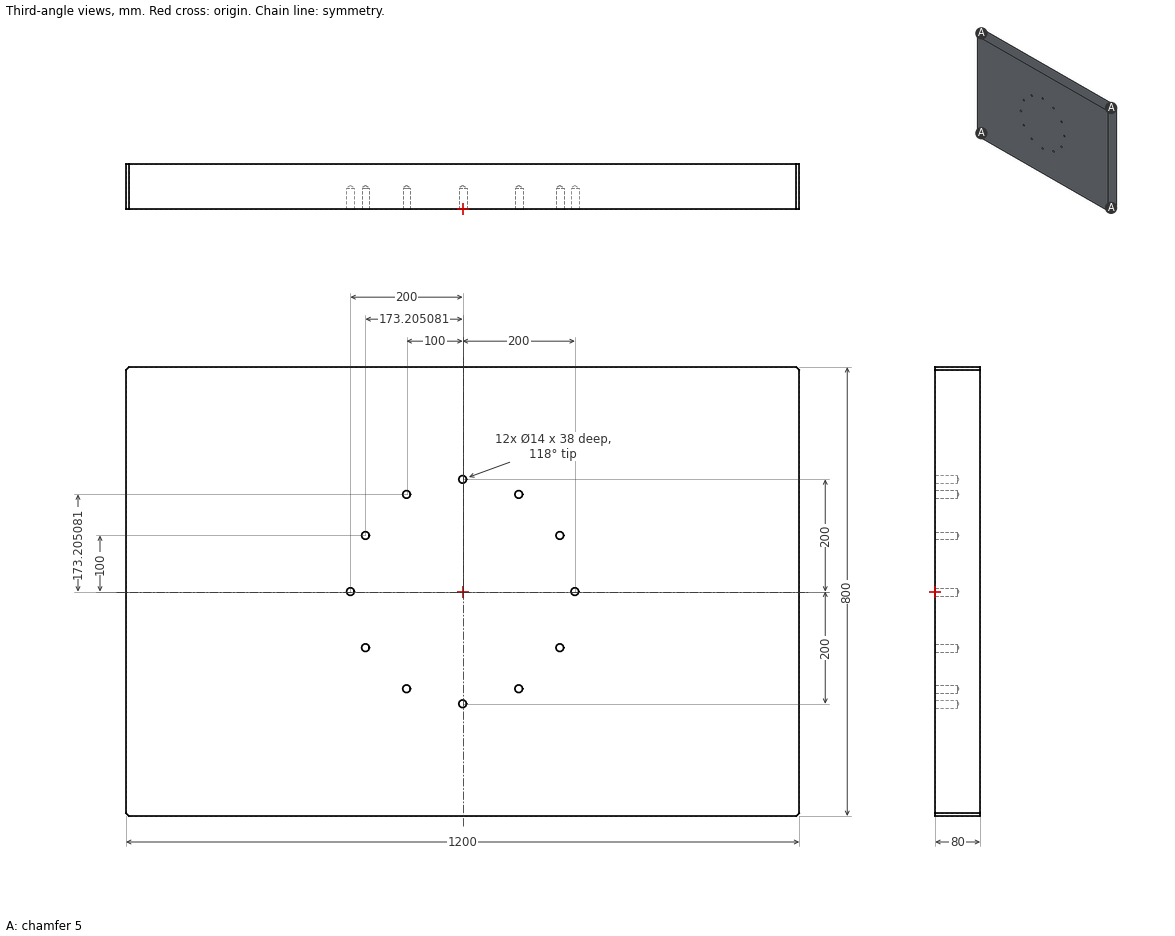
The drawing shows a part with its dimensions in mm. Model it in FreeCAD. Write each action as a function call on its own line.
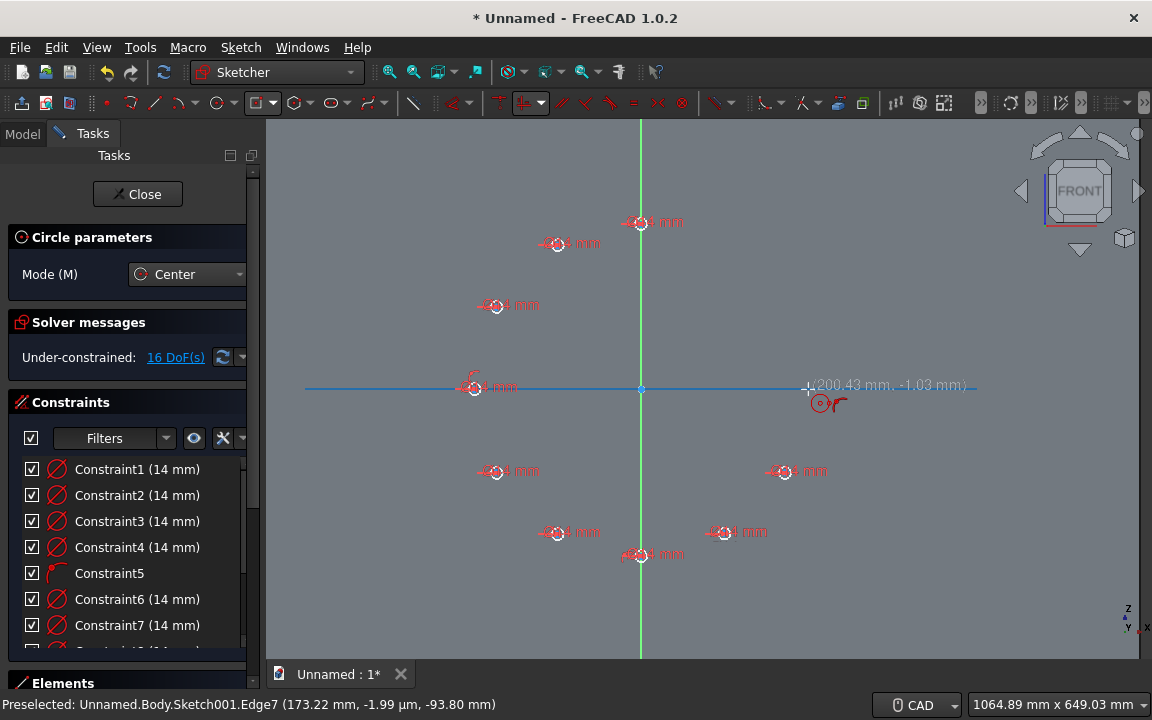
click(808, 389)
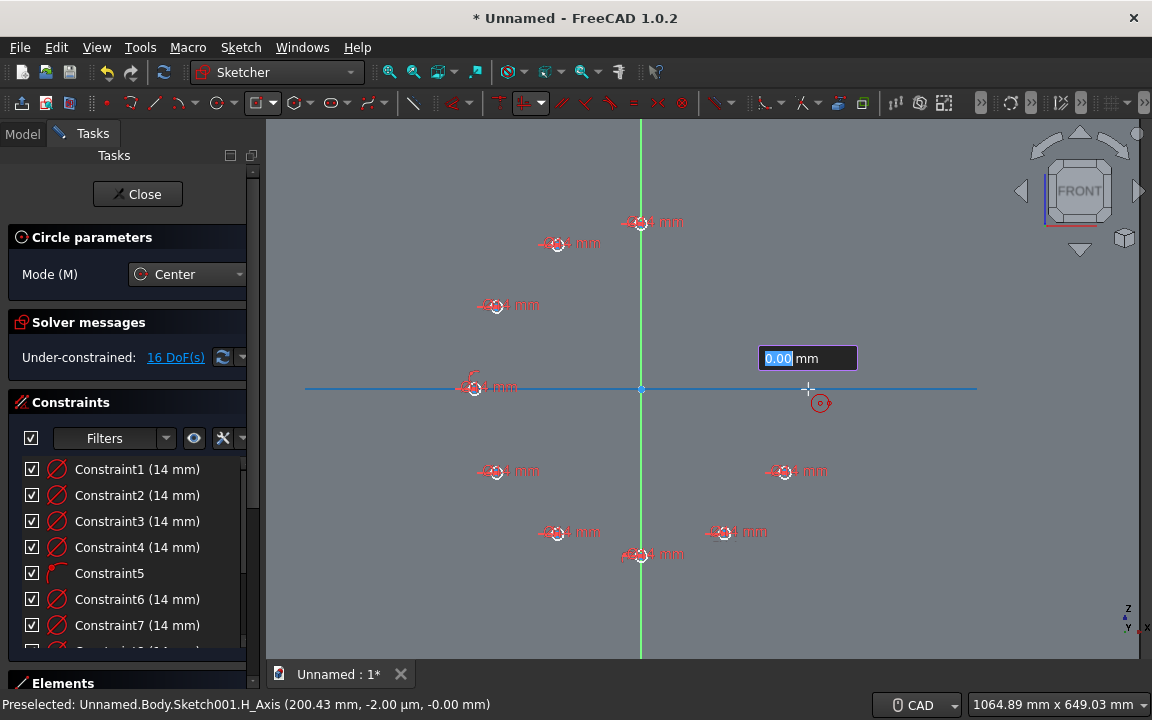
scroll(810, 384, up, 6)
move(807, 382)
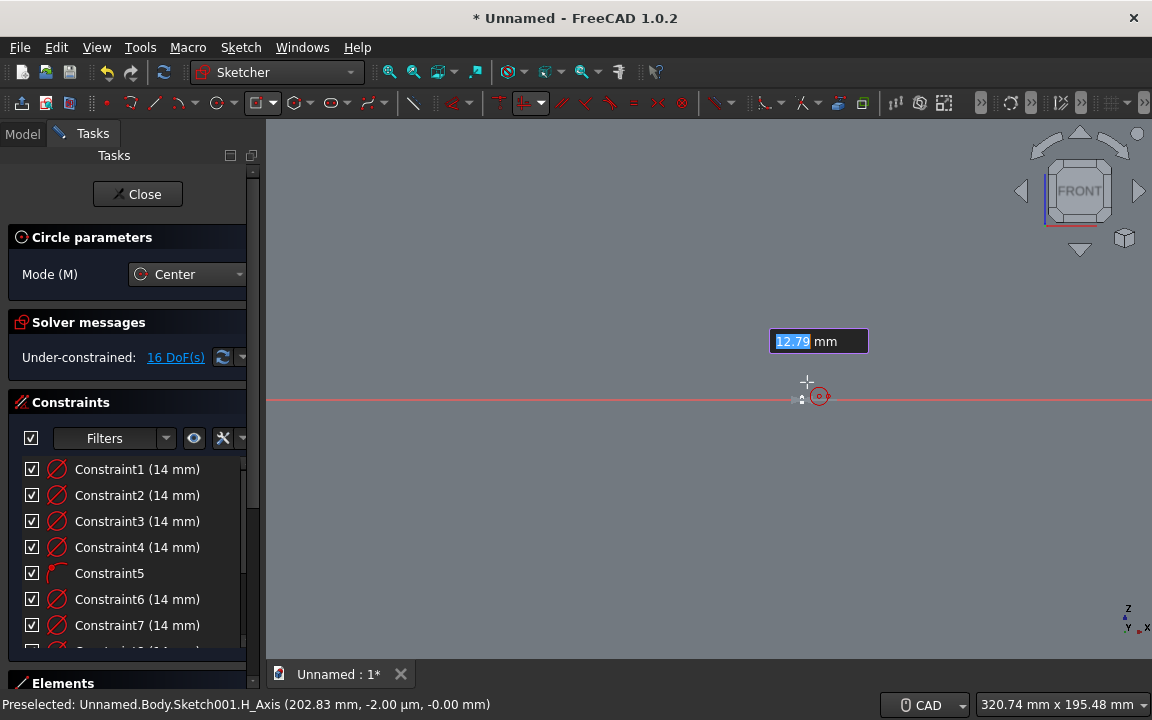
text(14)
key(Return)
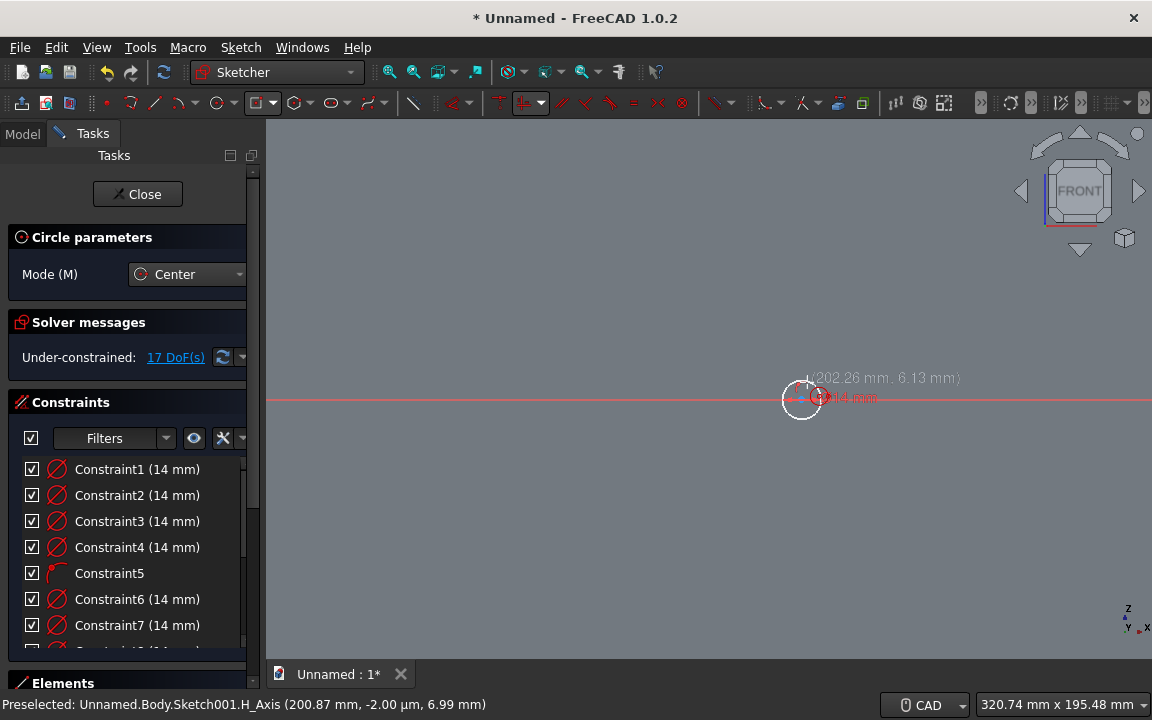
scroll(810, 384, down, 6)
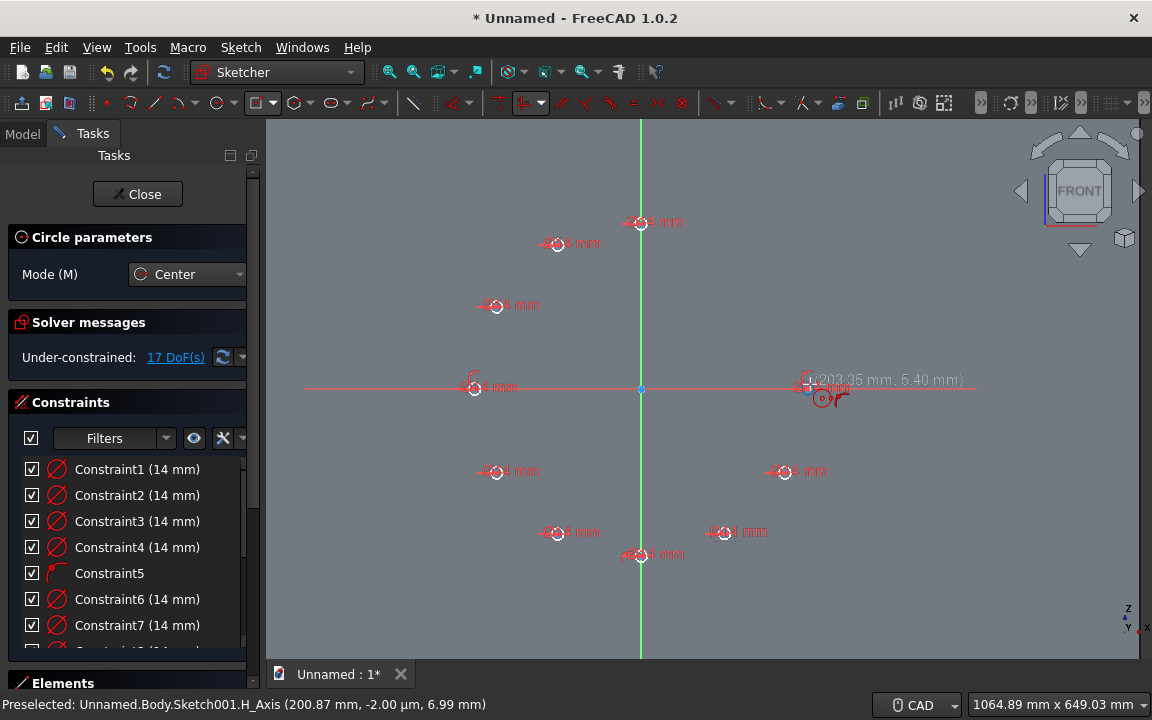
scroll(785, 306, up, 7)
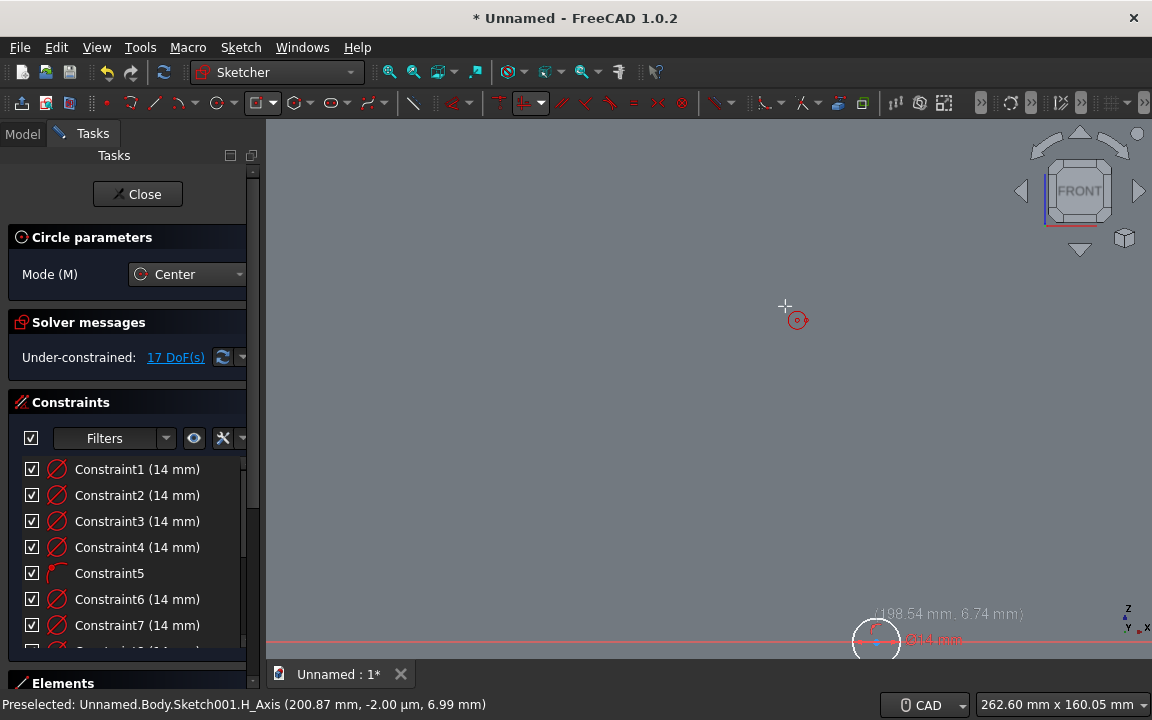
scroll(785, 306, down, 7)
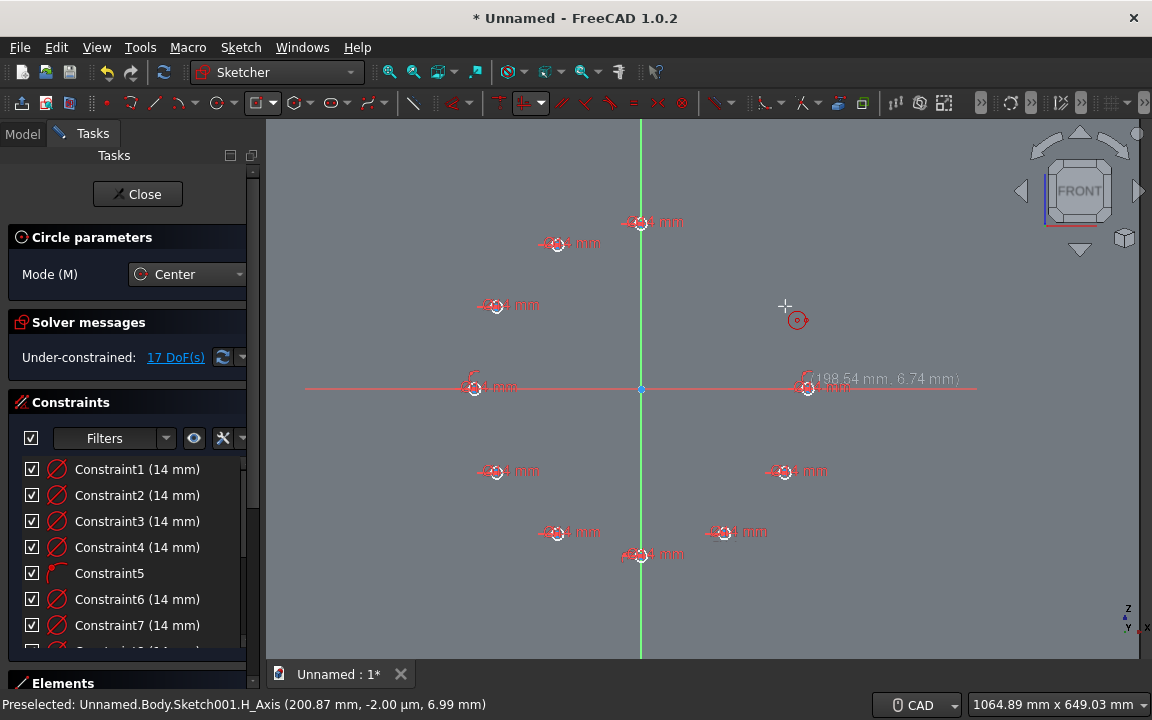
click(785, 306)
move(789, 302)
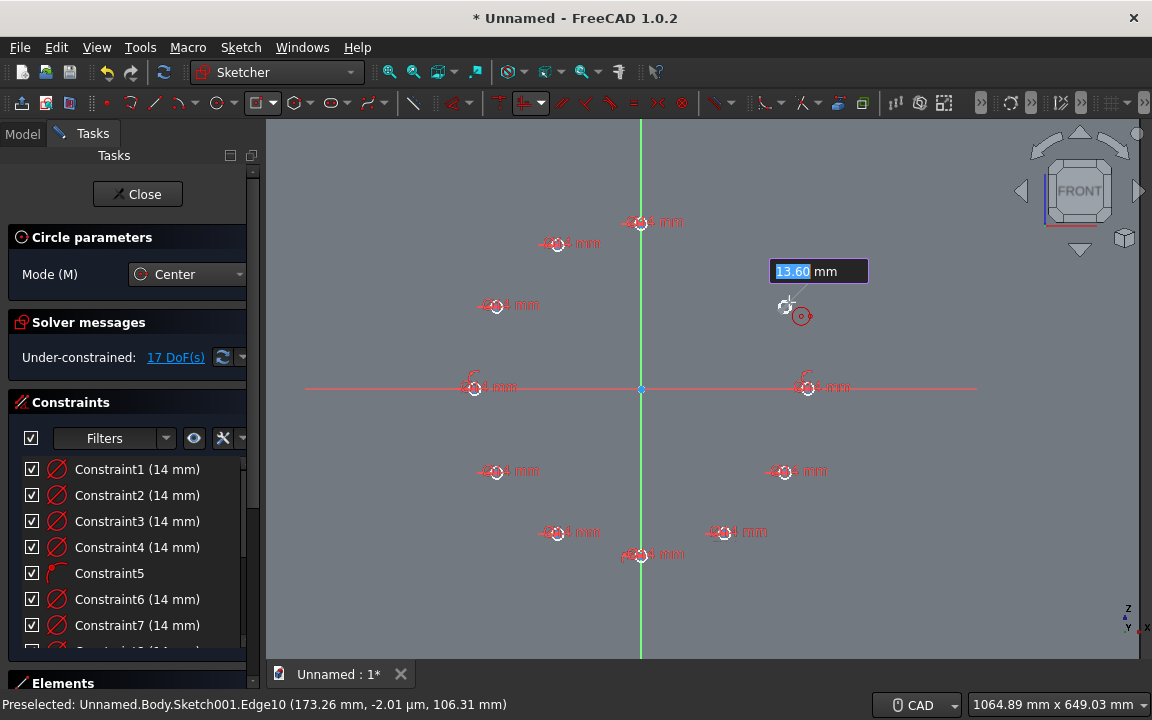
text(14)
key(Return)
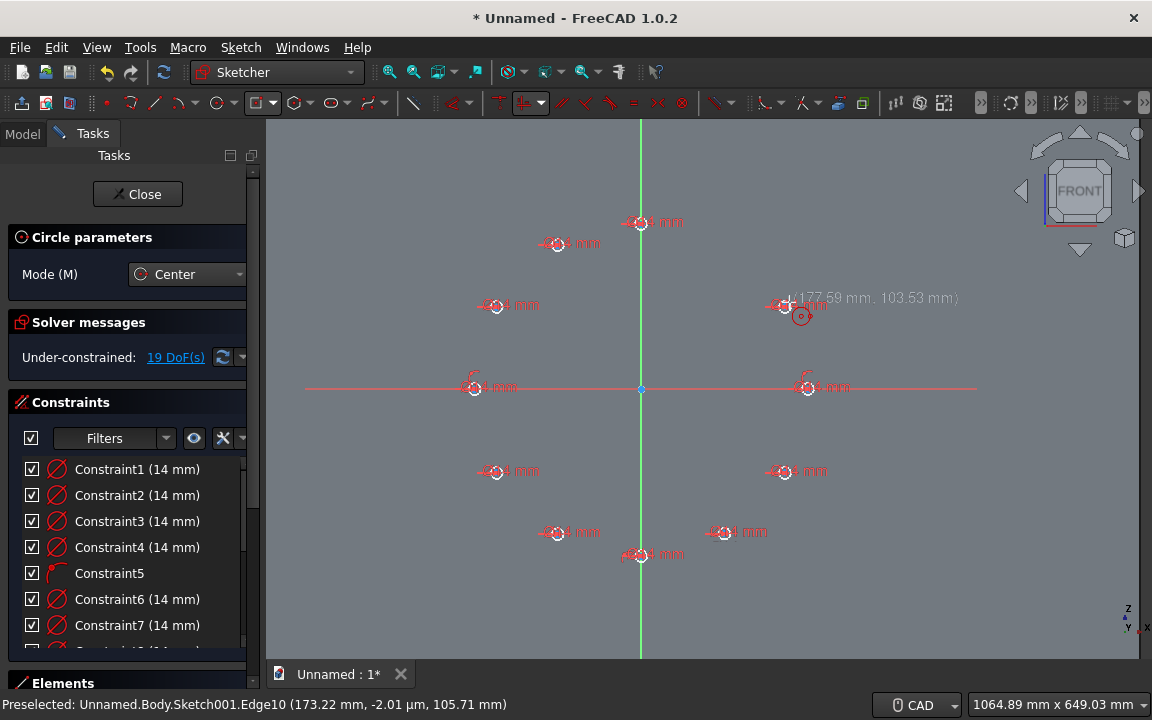
scroll(724, 245, up, 7)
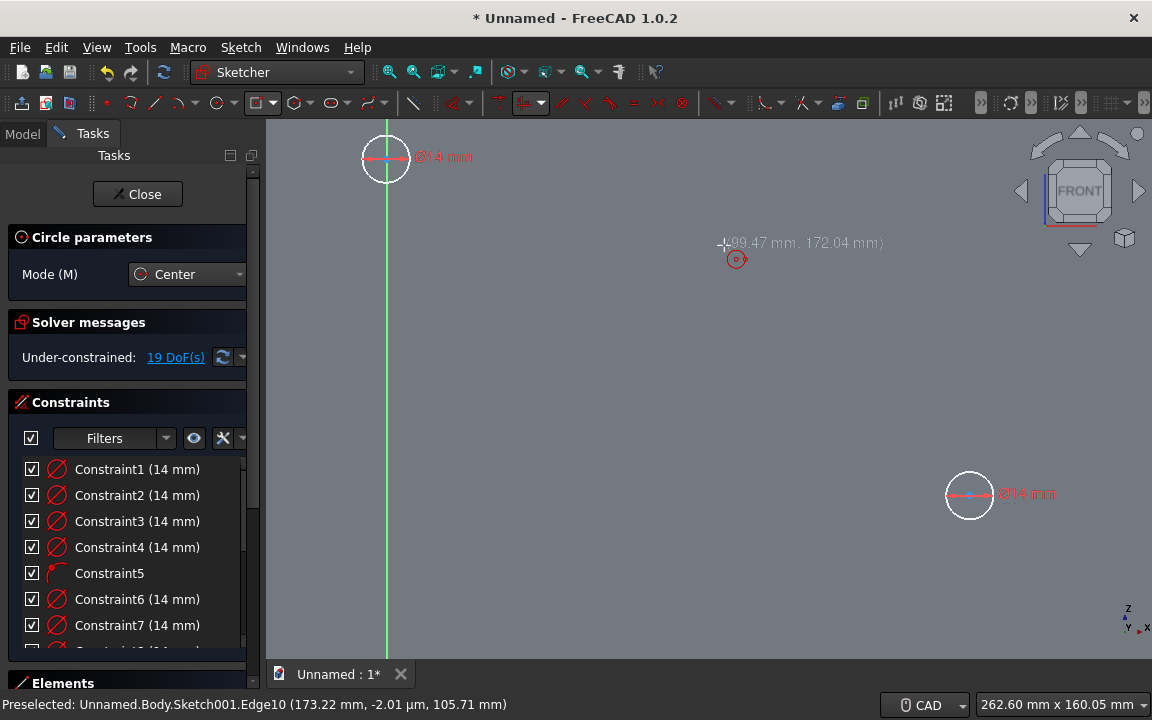
scroll(724, 245, down, 7)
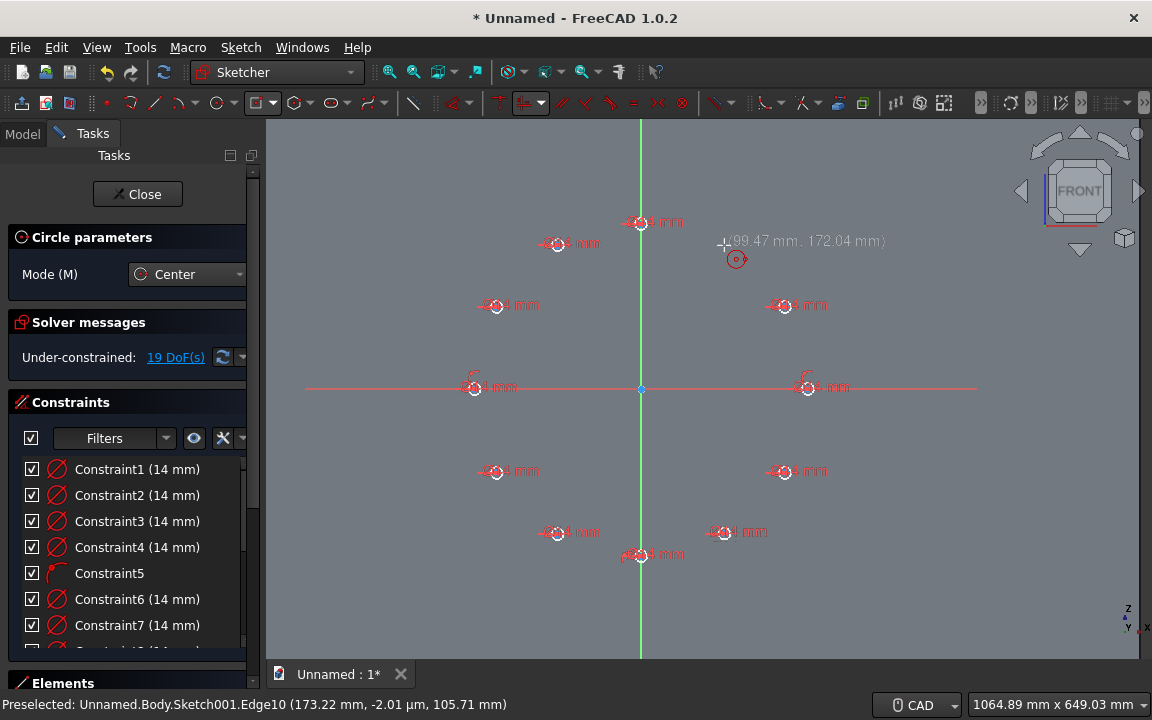
click(724, 245)
move(729, 241)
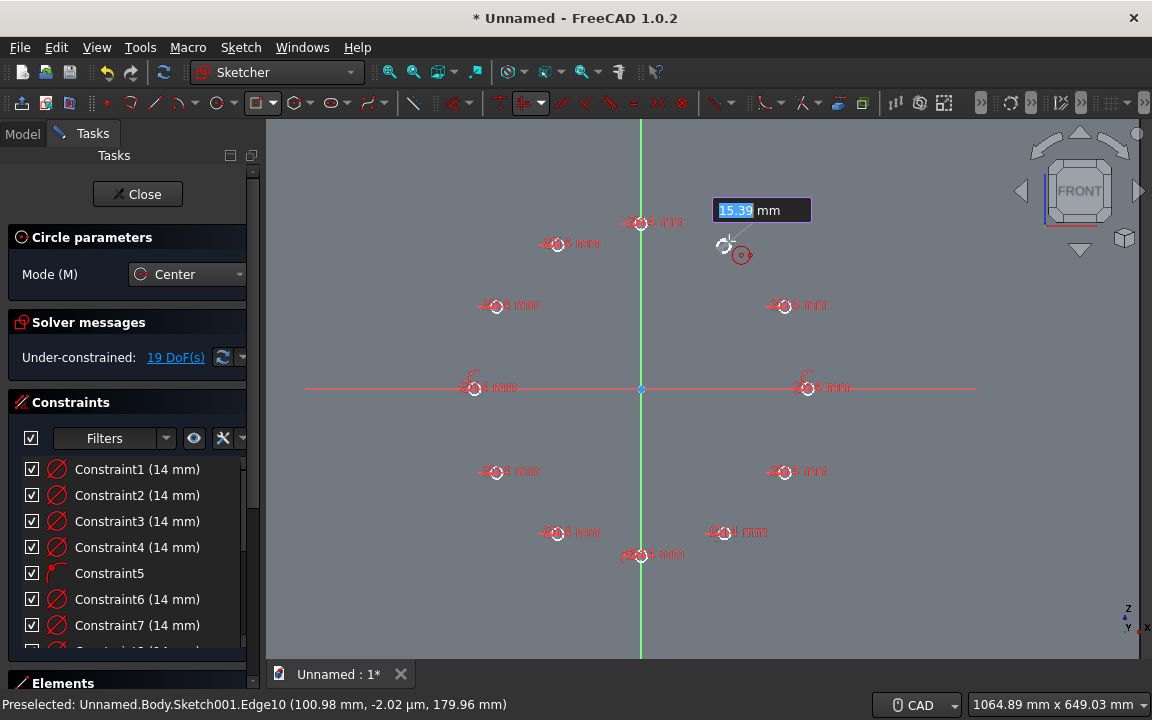
text(14)
key(Return)
key(Escape)